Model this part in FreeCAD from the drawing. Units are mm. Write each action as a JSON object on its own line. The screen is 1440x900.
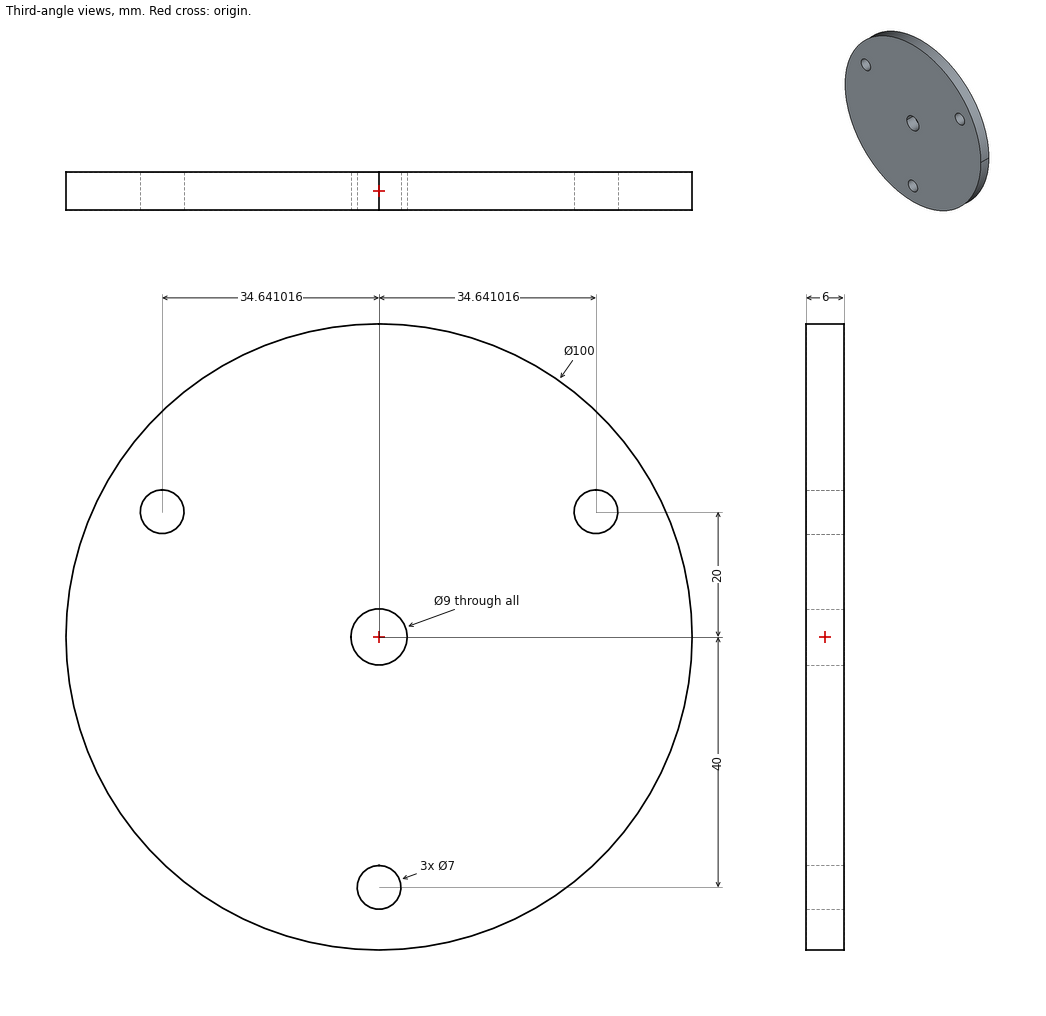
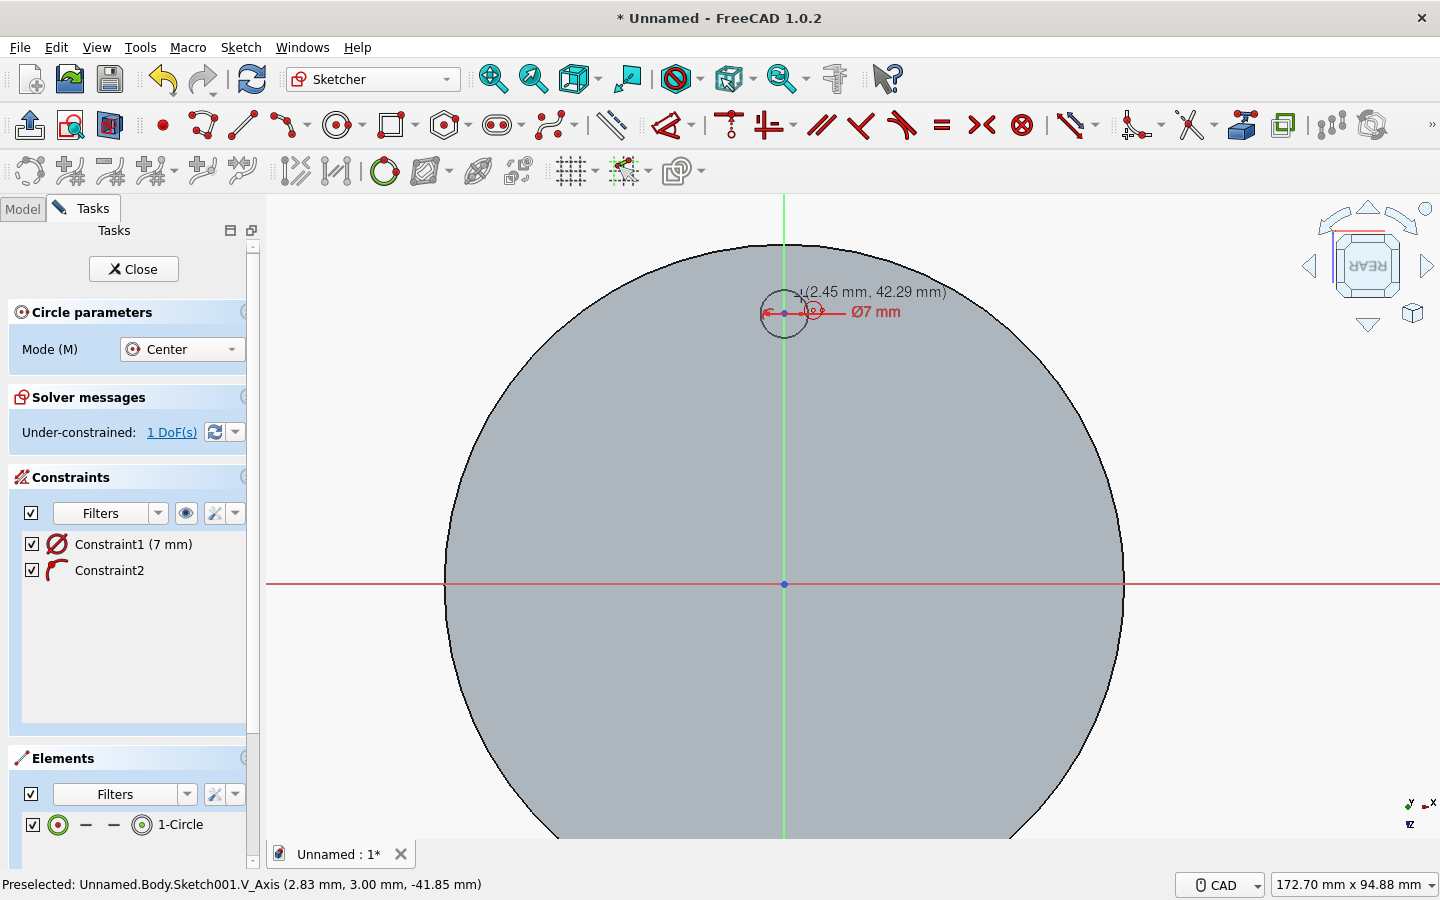
{"action": "left_click", "coordinate": [1020, 720]}
{"action": "mouse_move", "coordinate": [1037, 704]}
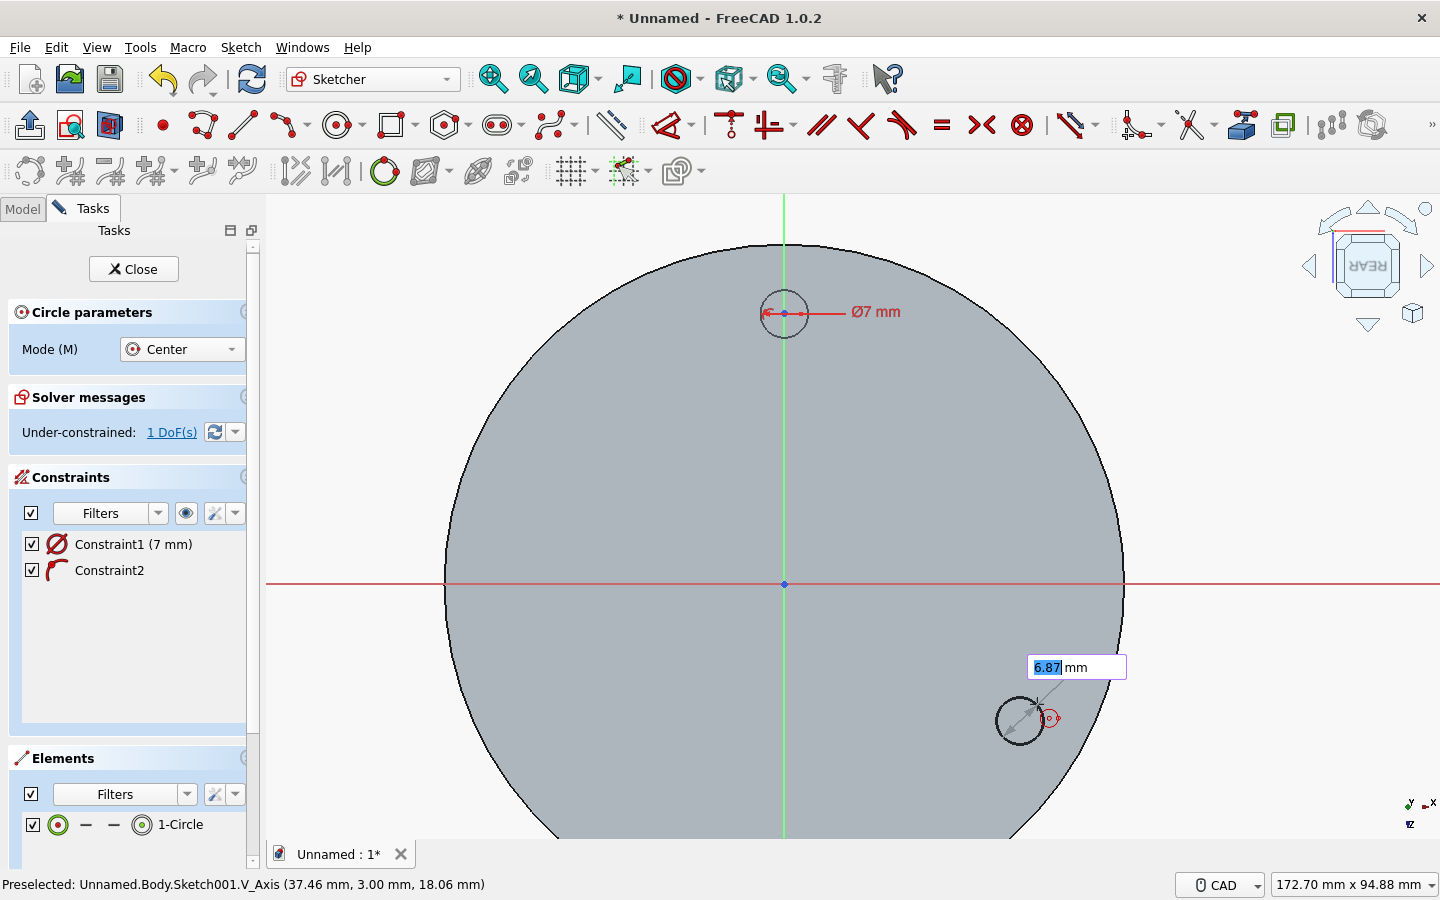
{"action": "type", "text": "7"}
{"action": "key", "text": "Return"}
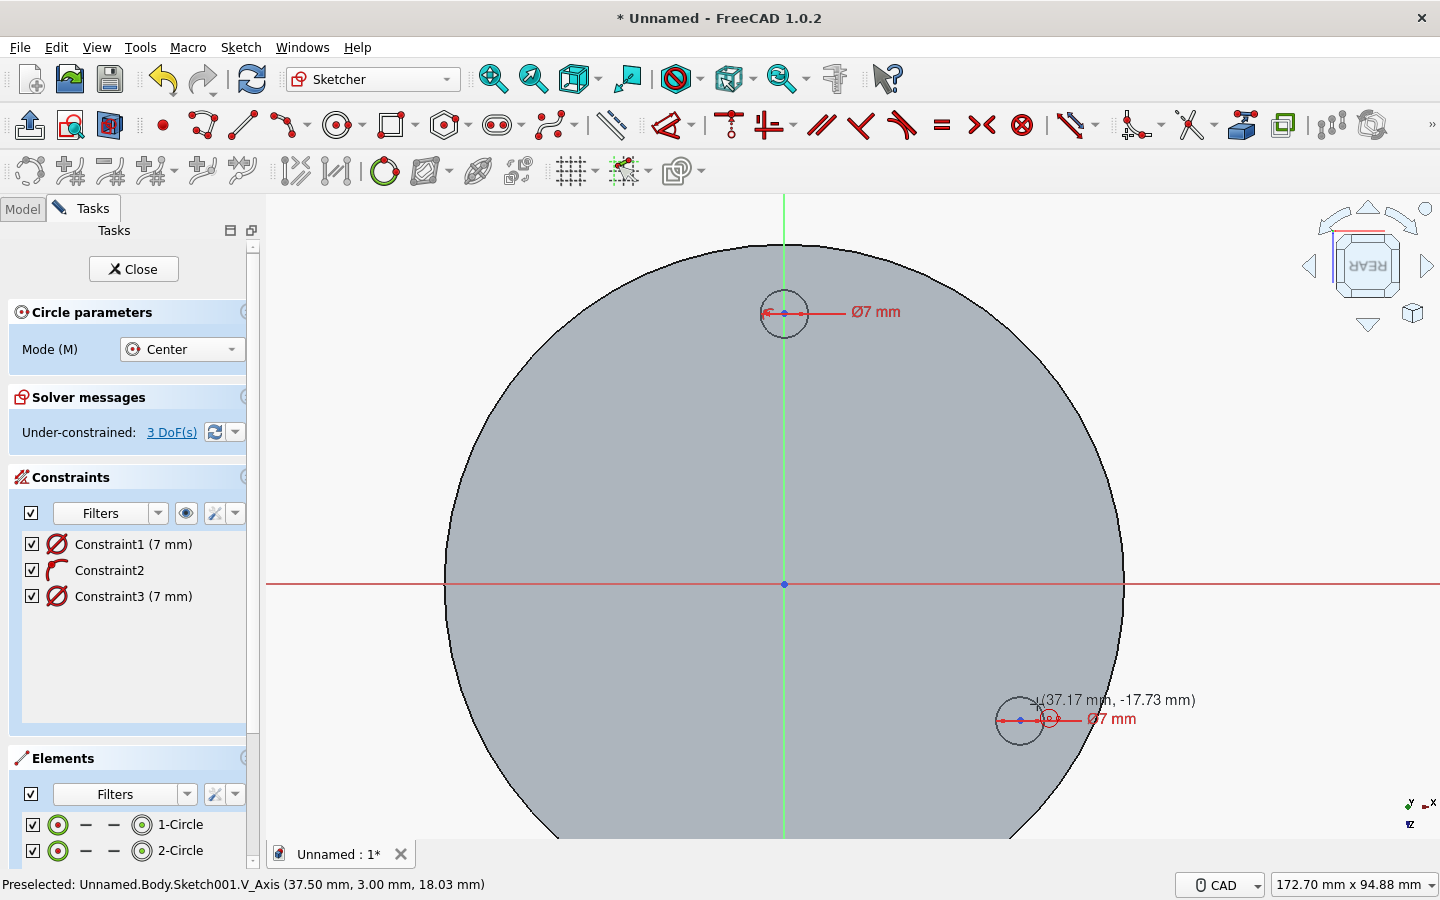
{"action": "left_click", "coordinate": [549, 720]}
{"action": "mouse_move", "coordinate": [566, 704]}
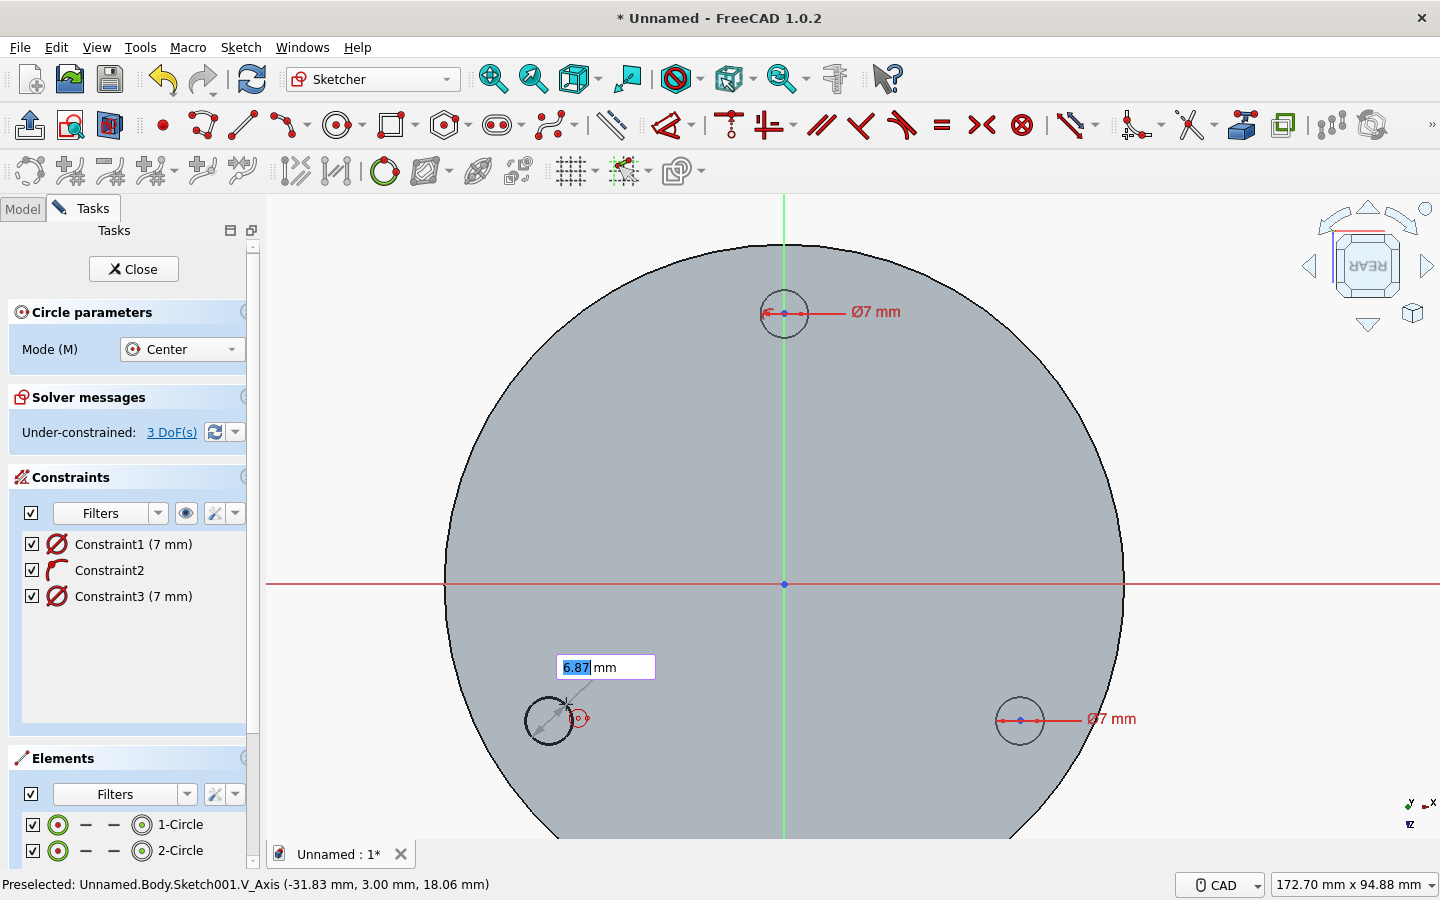
{"action": "type", "text": "7"}
{"action": "key", "text": "Return"}
{"action": "key", "text": "Escape"}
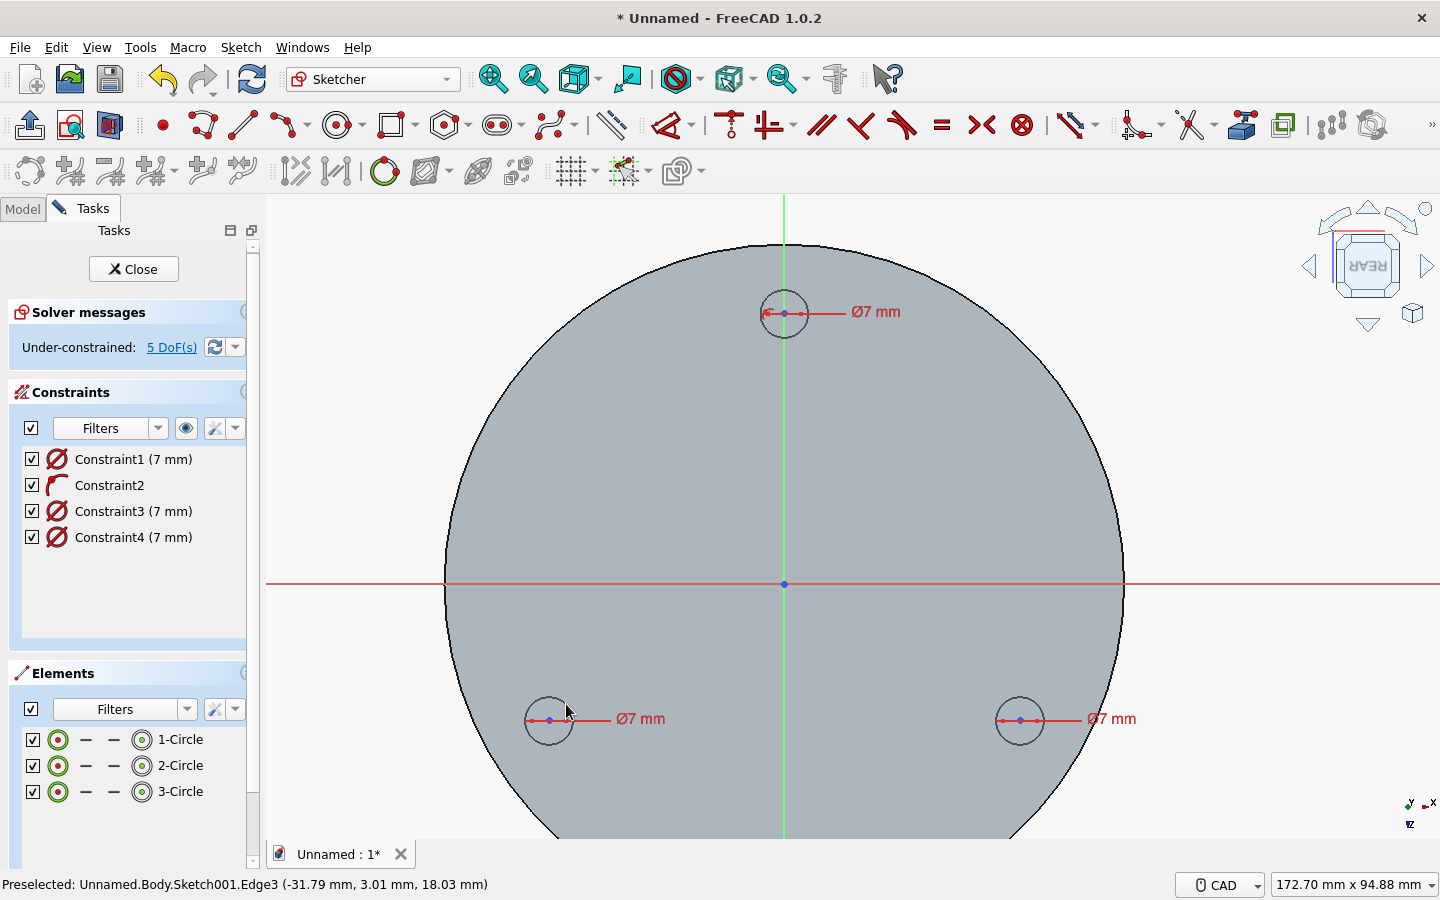
{"action": "left_click", "coordinate": [1020, 721]}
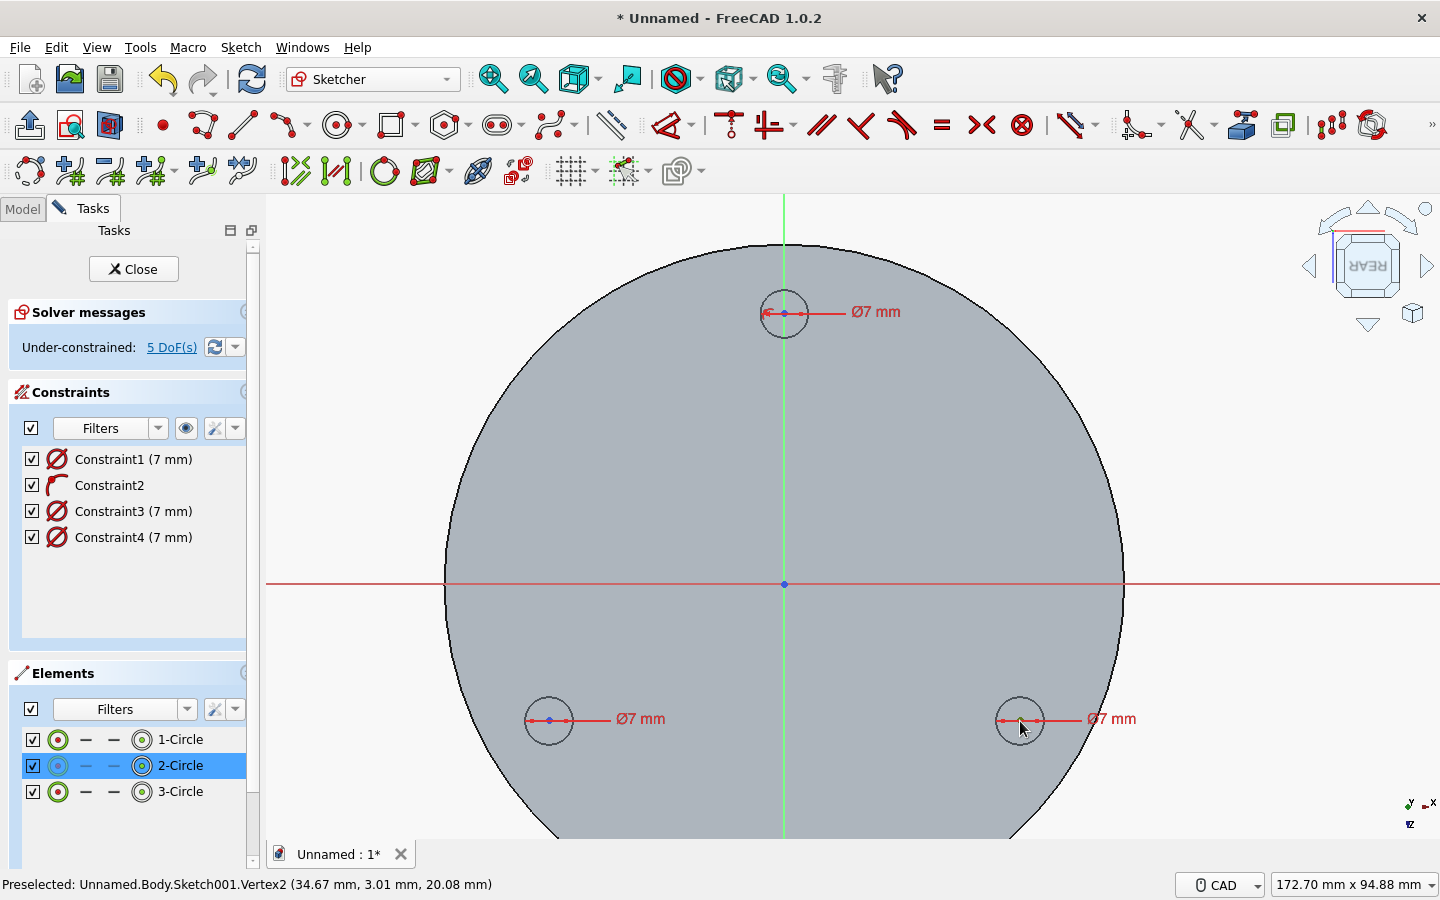
{"action": "left_click", "coordinate": [549, 721]}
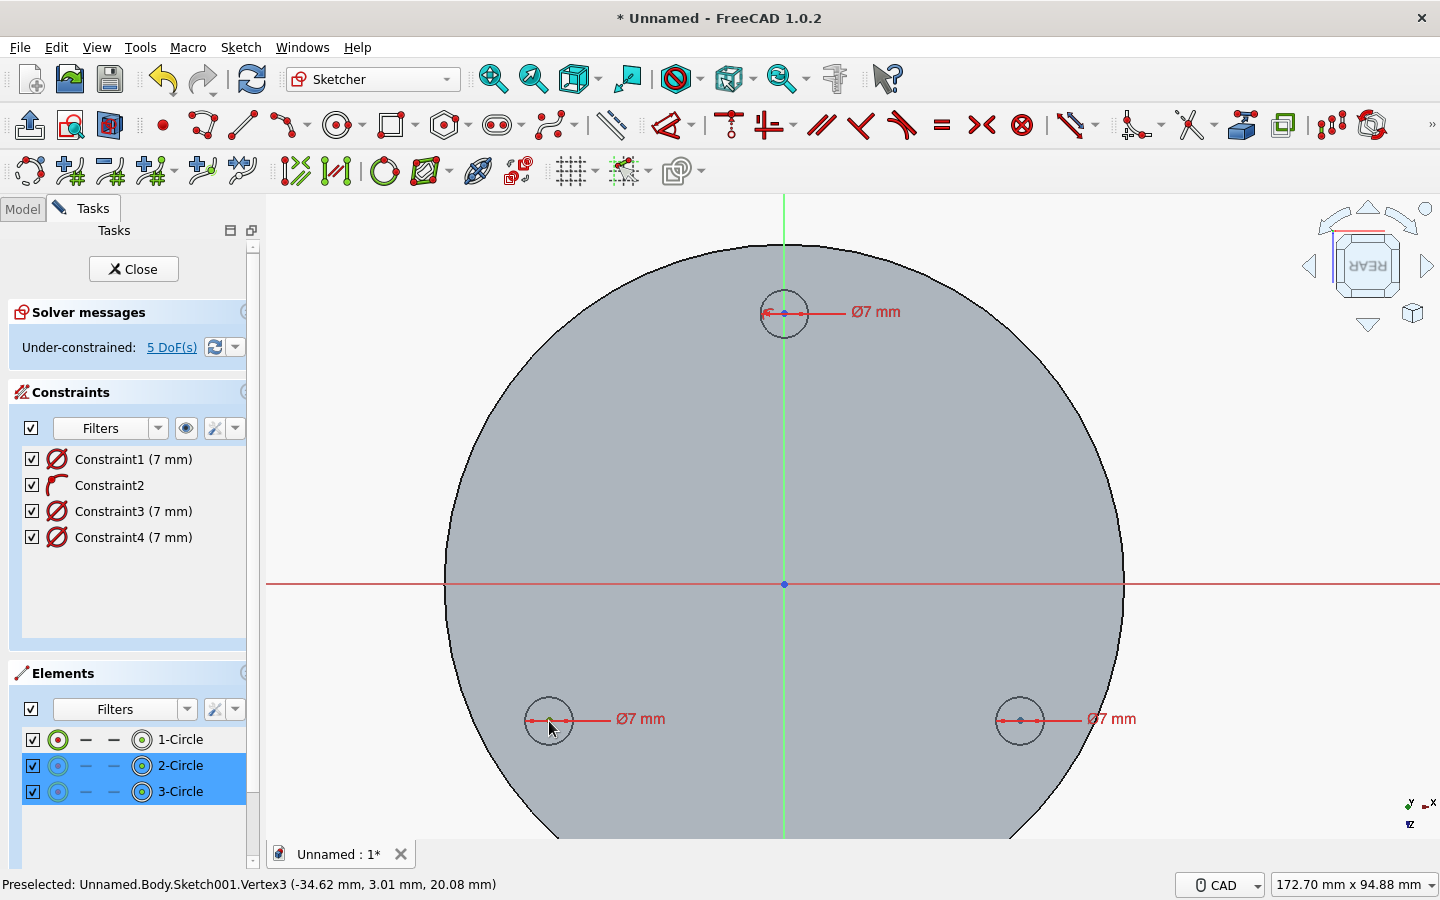
{"action": "key", "text": "h"}